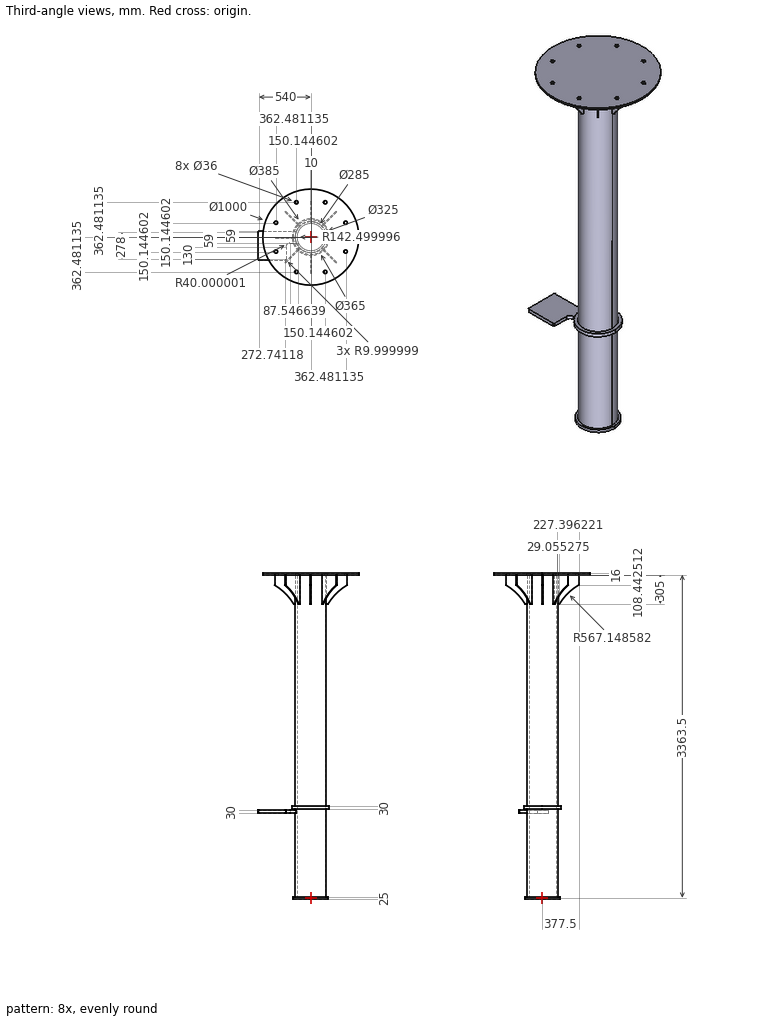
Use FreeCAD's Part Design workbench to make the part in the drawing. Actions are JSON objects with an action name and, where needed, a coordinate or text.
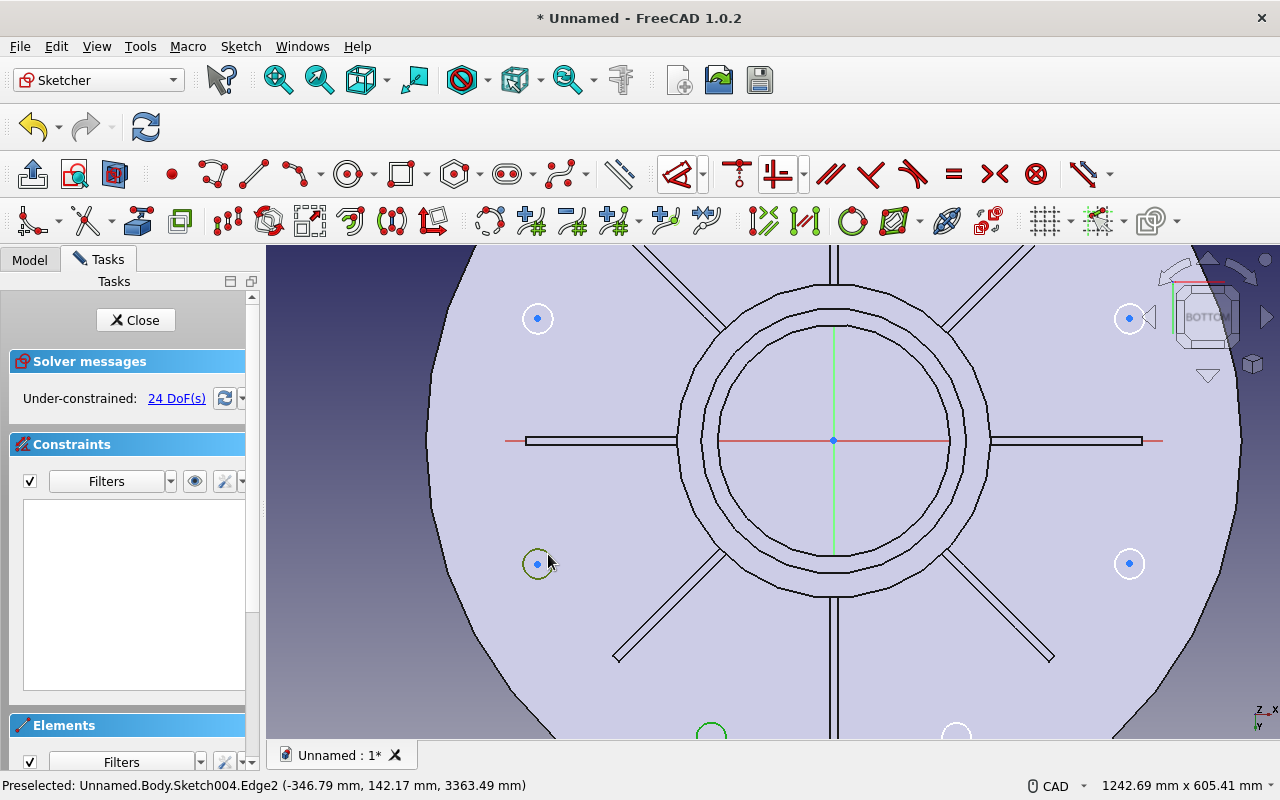
{"action": "left_click", "coordinate": [548, 308]}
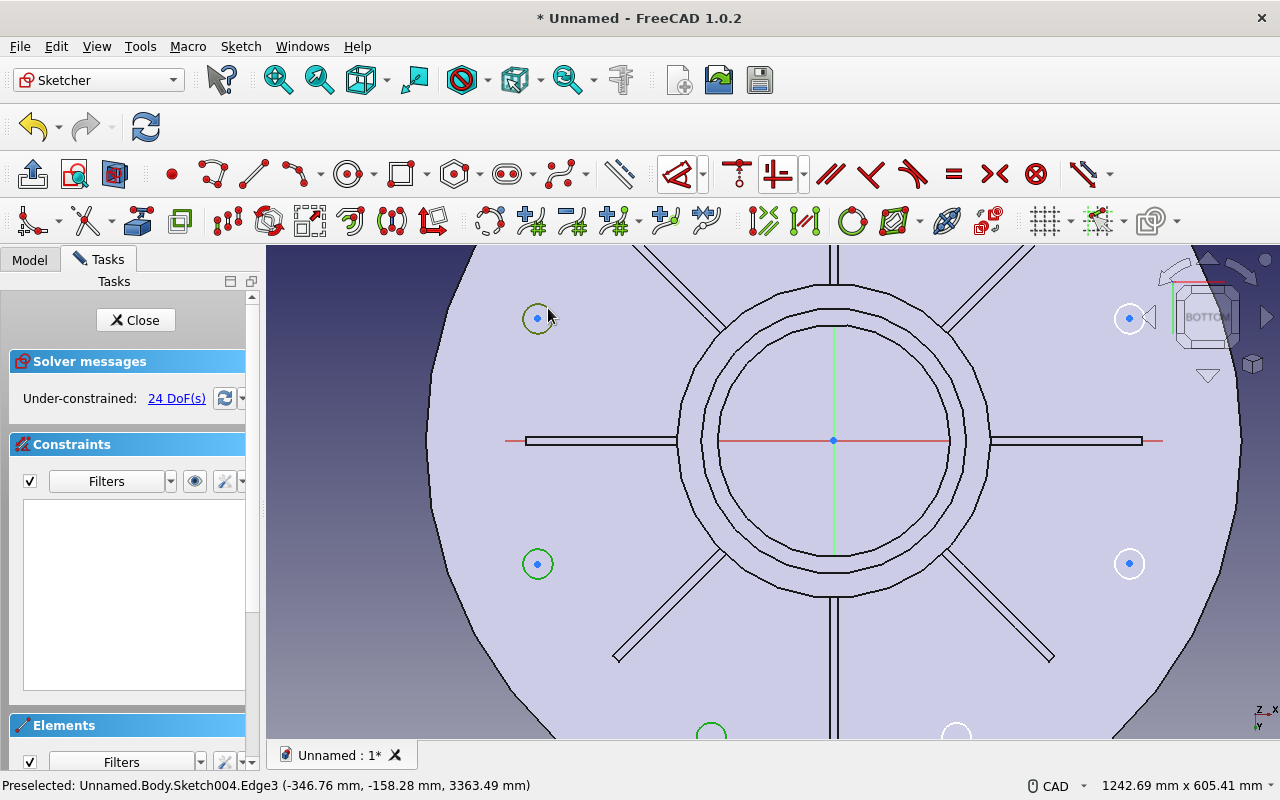
{"action": "scroll", "coordinate": [547, 554], "scroll_direction": "down", "scroll_amount": 3}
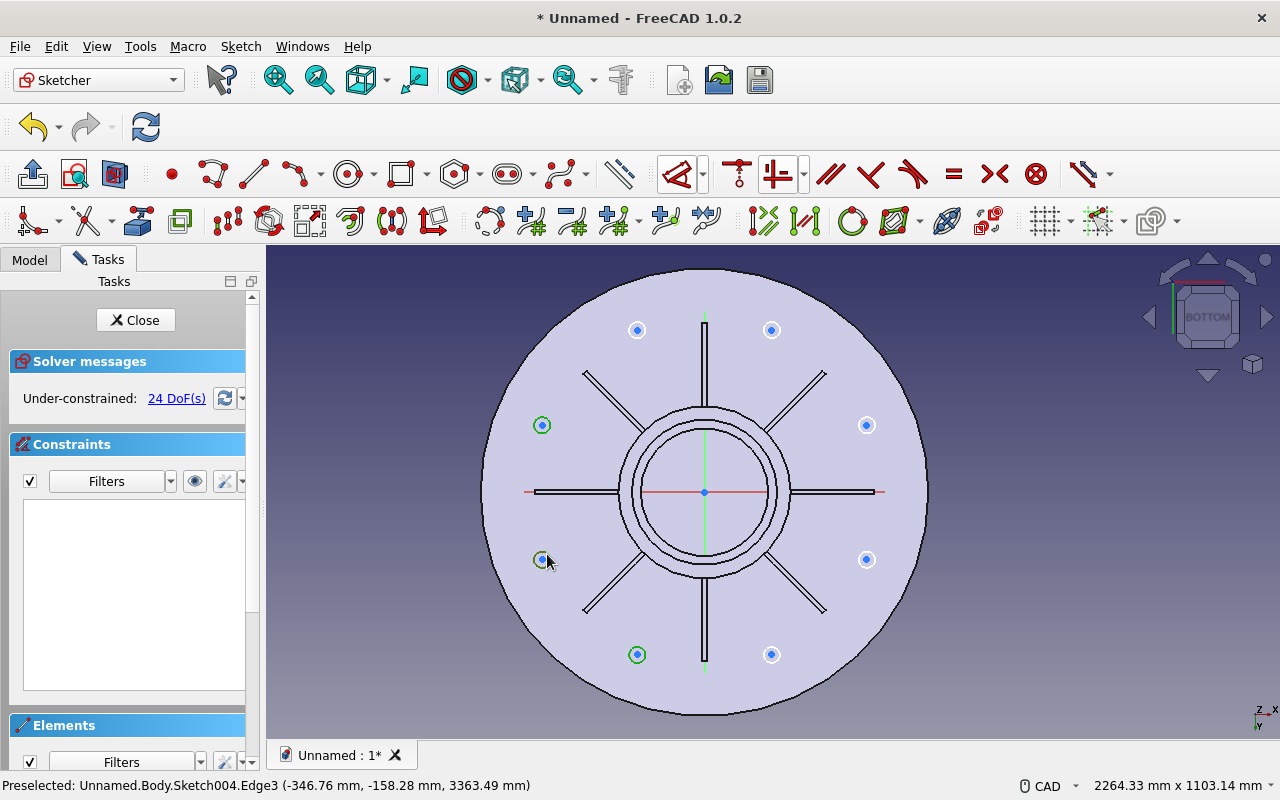
{"action": "scroll", "coordinate": [643, 324], "scroll_direction": "up", "scroll_amount": 3}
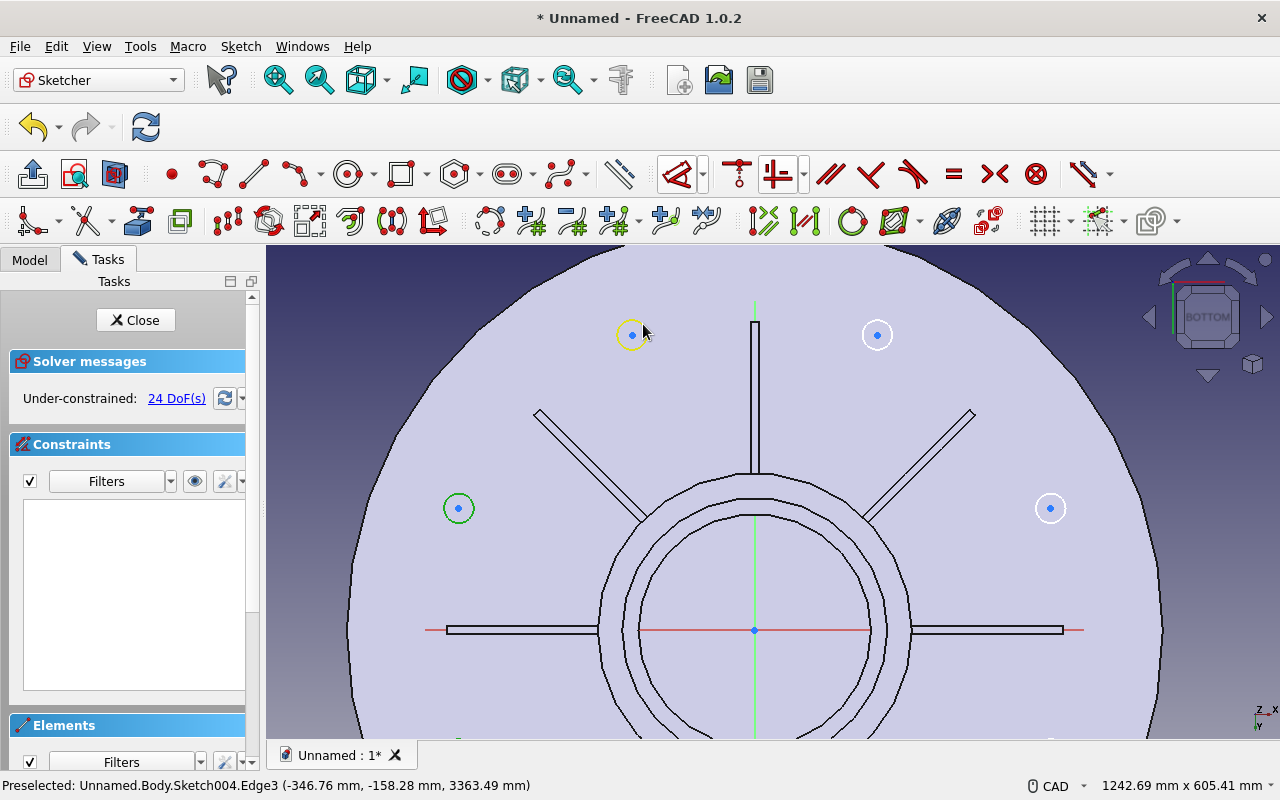
{"action": "left_click", "coordinate": [643, 325]}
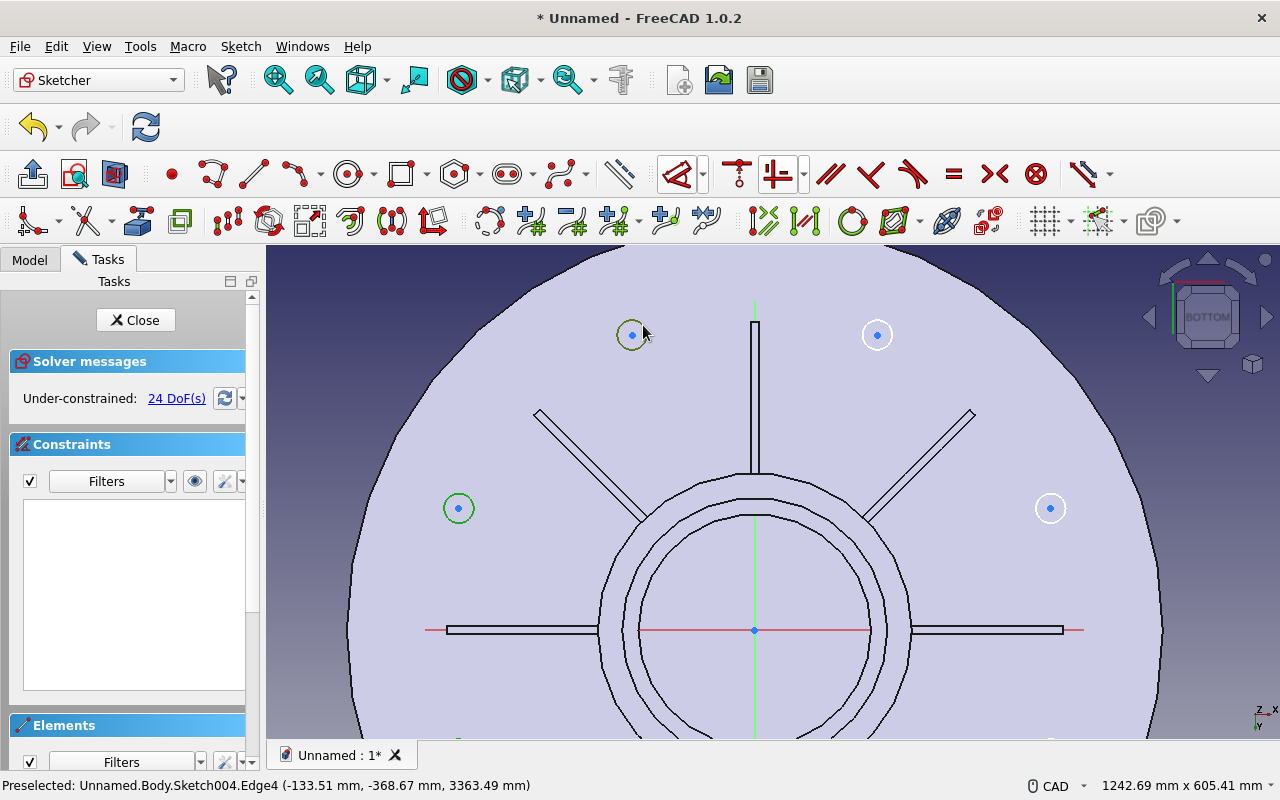
{"action": "left_click", "coordinate": [888, 325]}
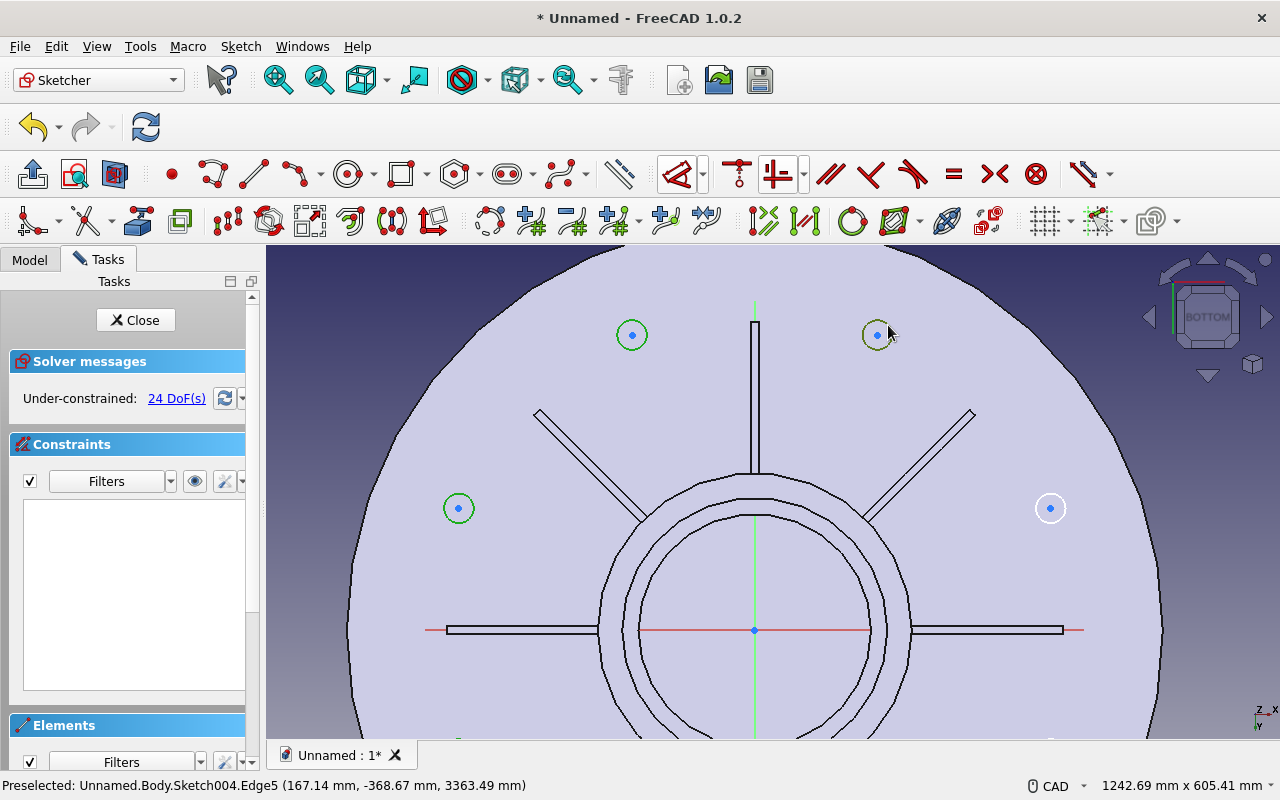
{"action": "left_click", "coordinate": [1061, 498]}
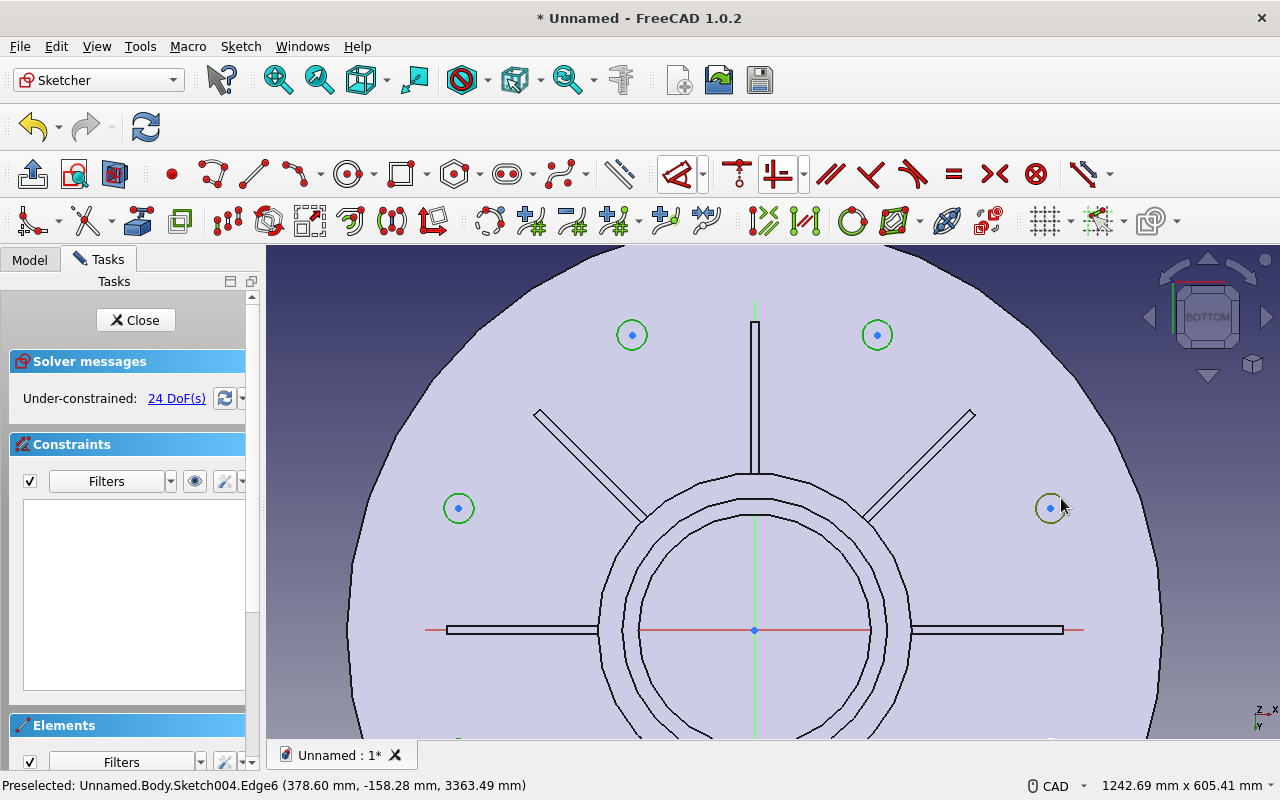
{"action": "scroll", "coordinate": [643, 324], "scroll_direction": "down", "scroll_amount": 3}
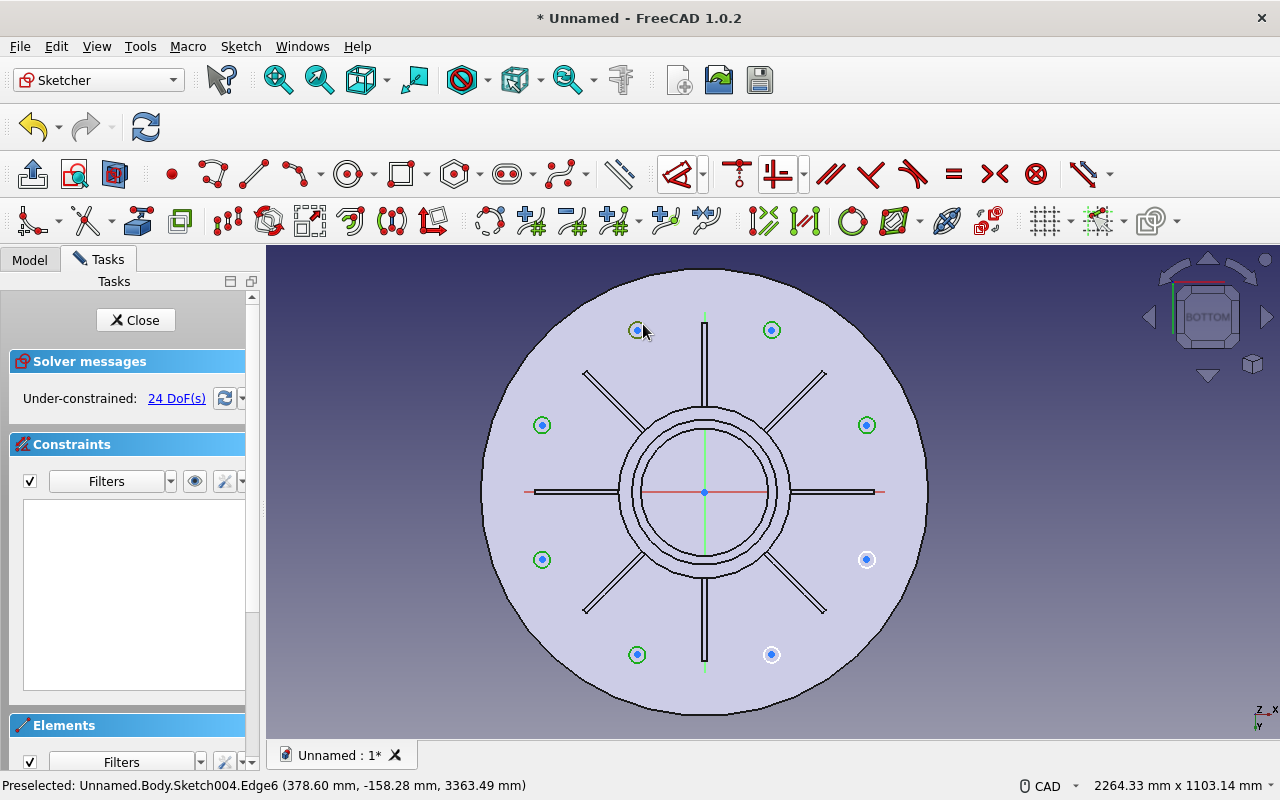
{"action": "scroll", "coordinate": [873, 554], "scroll_direction": "up", "scroll_amount": 3}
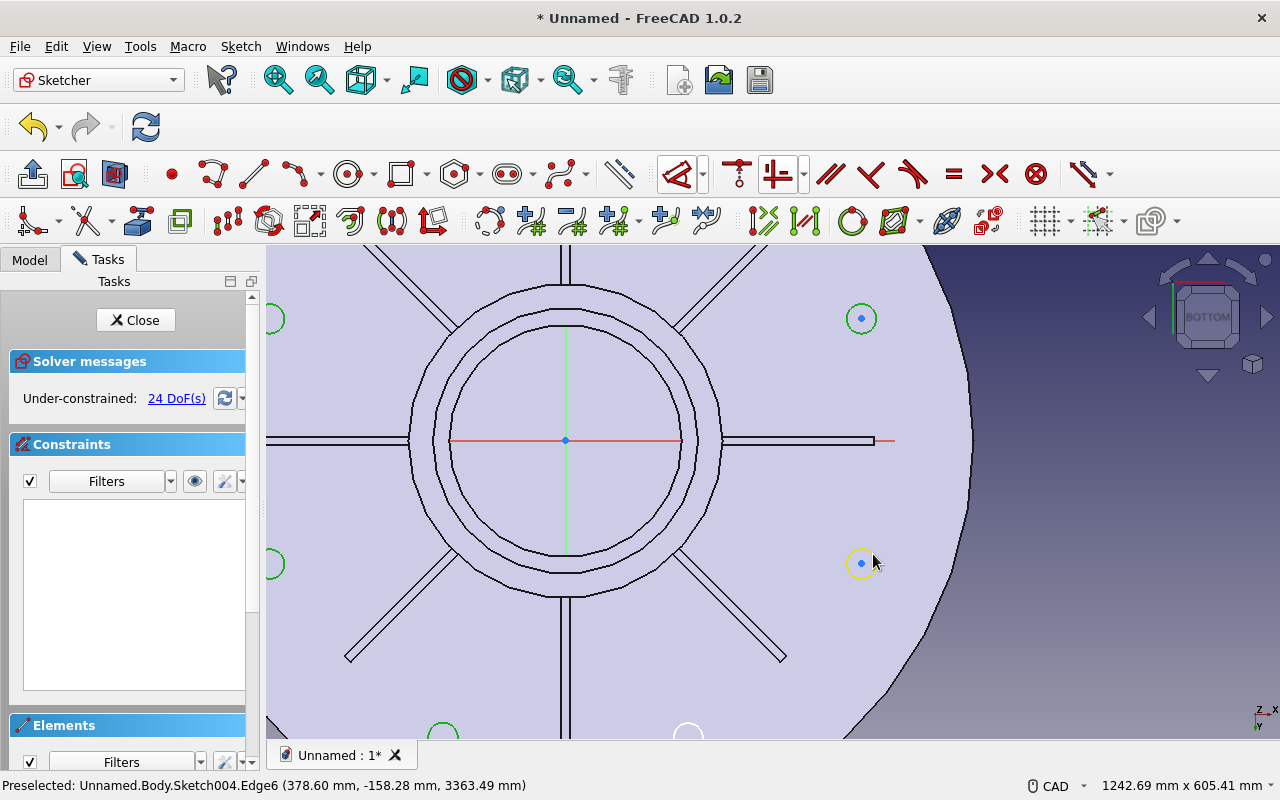
{"action": "left_click", "coordinate": [872, 553]}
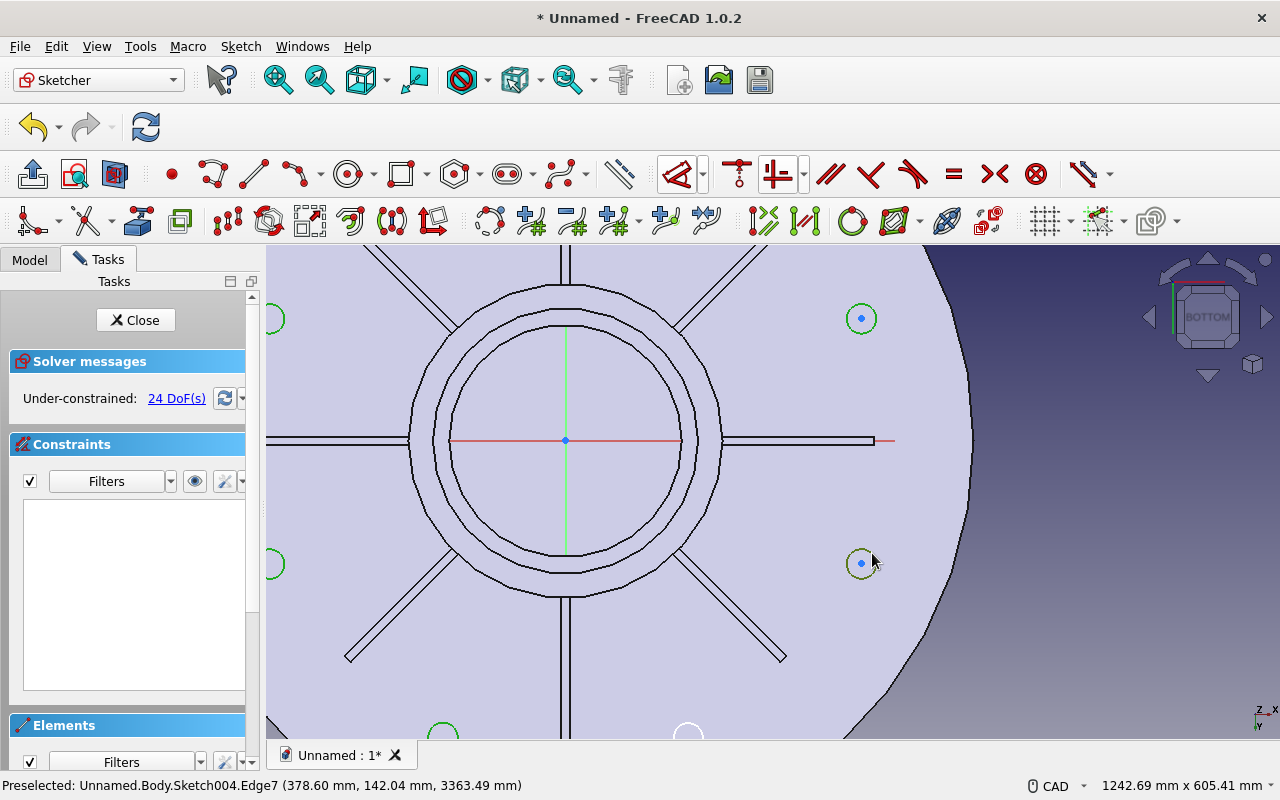
{"action": "scroll", "coordinate": [874, 554], "scroll_direction": "down", "scroll_amount": 3}